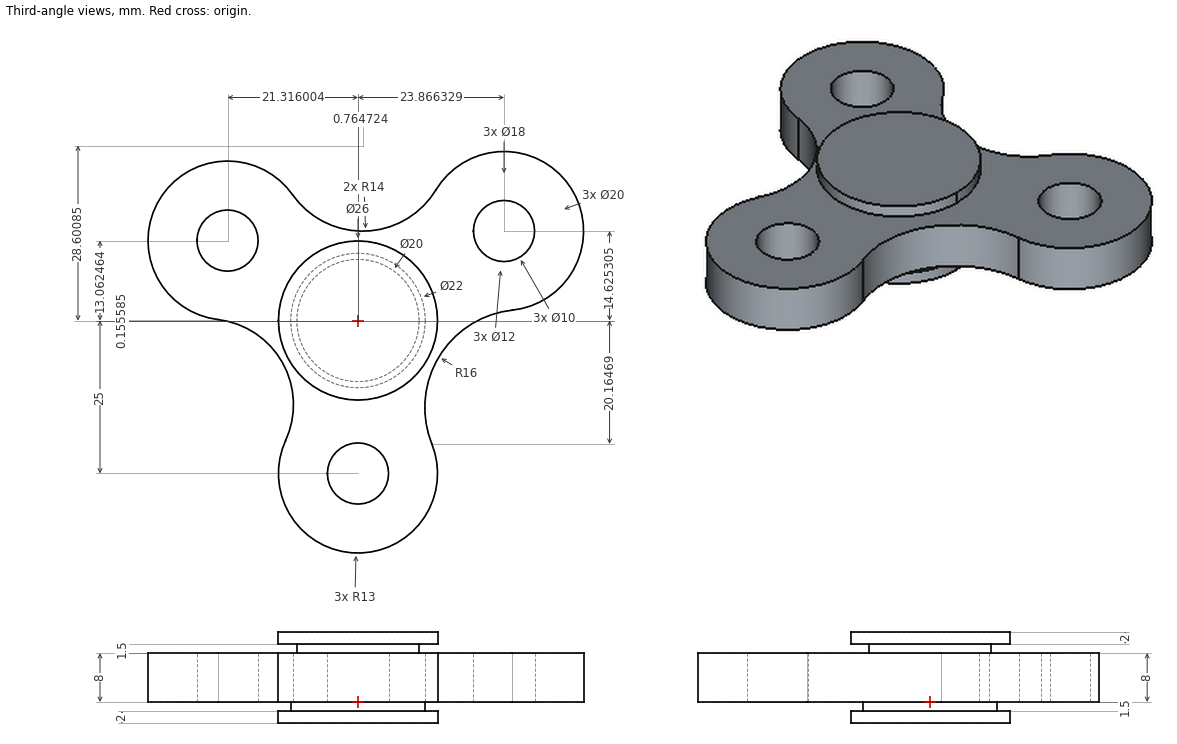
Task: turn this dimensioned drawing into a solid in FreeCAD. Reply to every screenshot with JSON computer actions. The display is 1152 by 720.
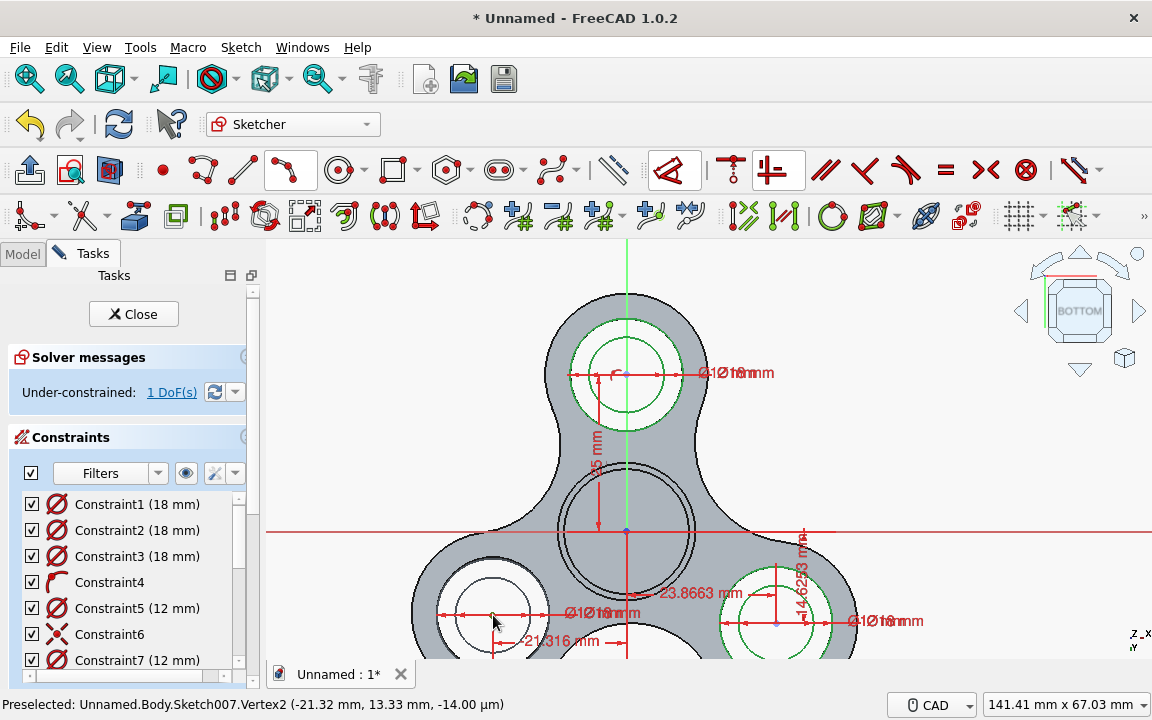
{"action": "key", "text": "i"}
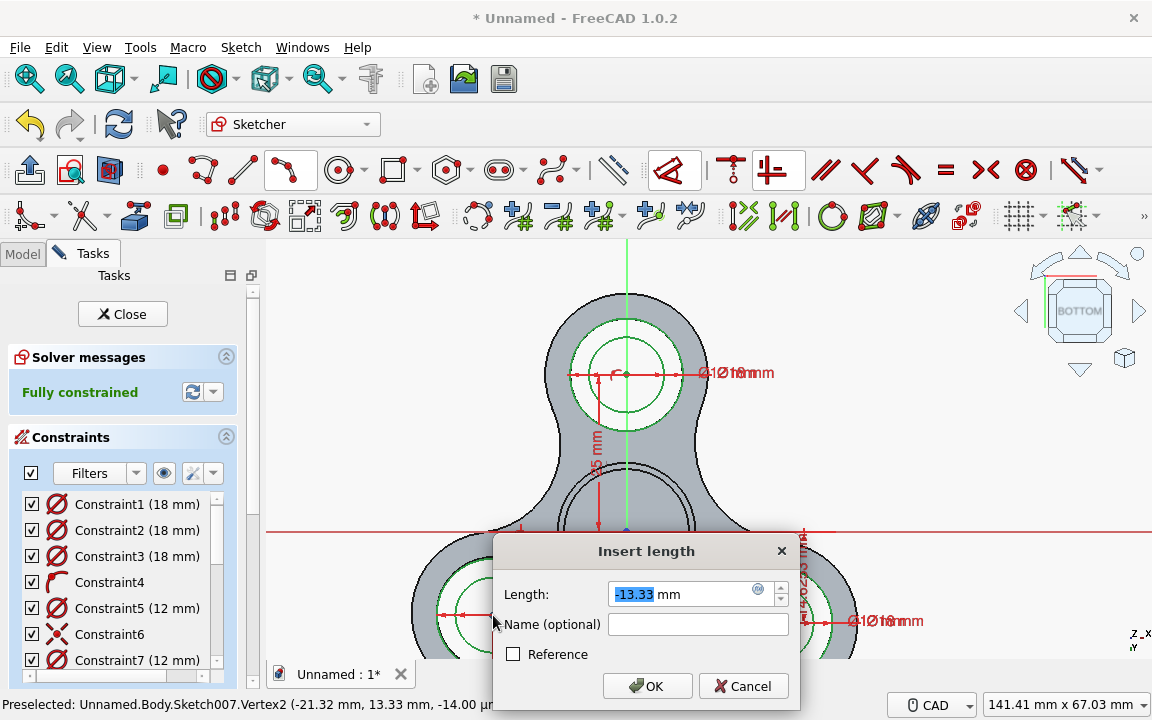
{"action": "type", "text": "-13.062464"}
{"action": "key", "text": "Return"}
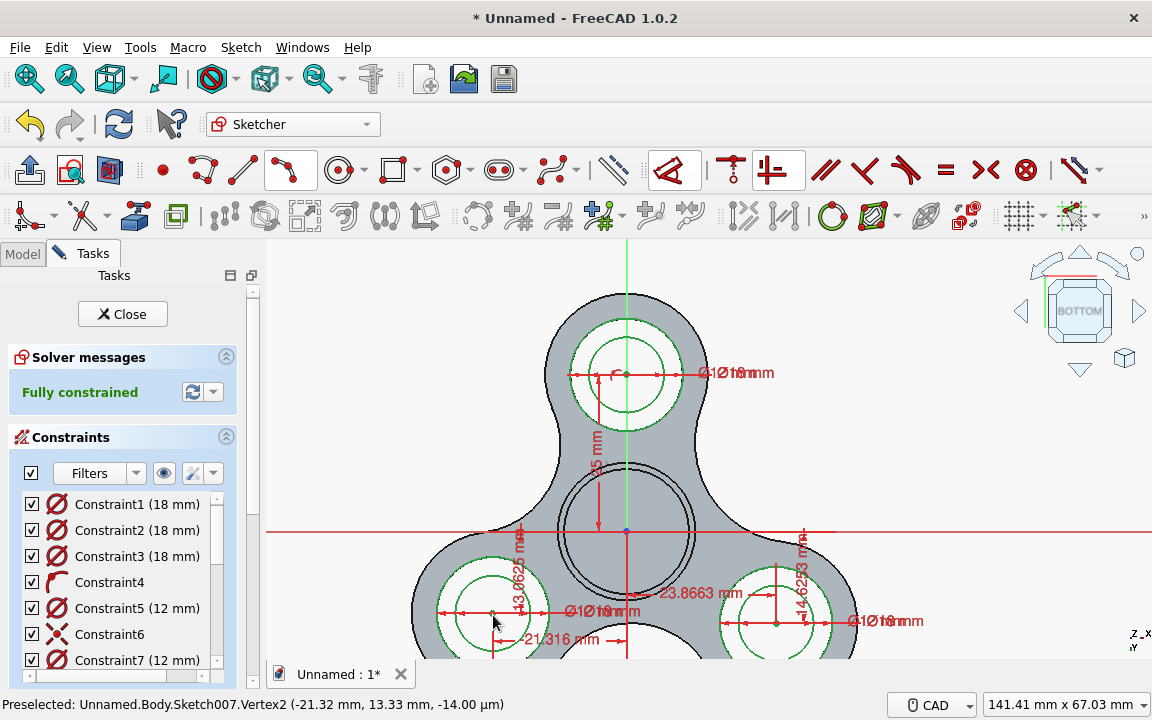
{"action": "left_click", "coordinate": [123, 314]}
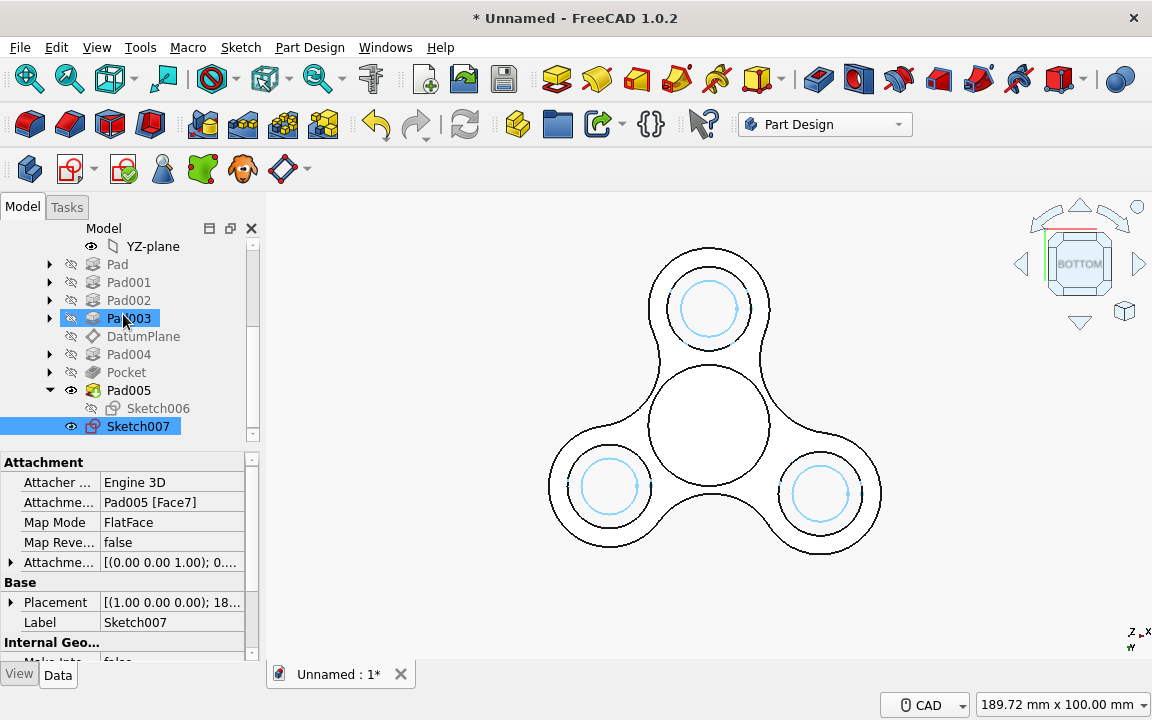
{"action": "left_click", "coordinate": [558, 80]}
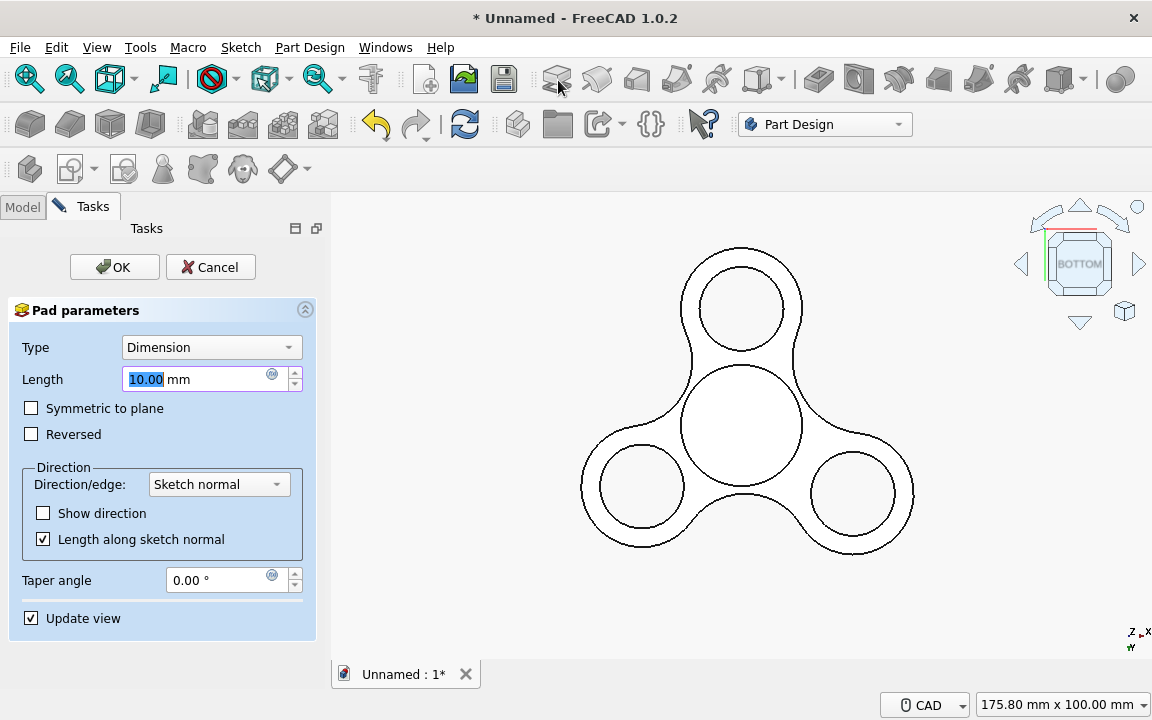
{"action": "type", "text": "8"}
{"action": "key", "text": "Tab"}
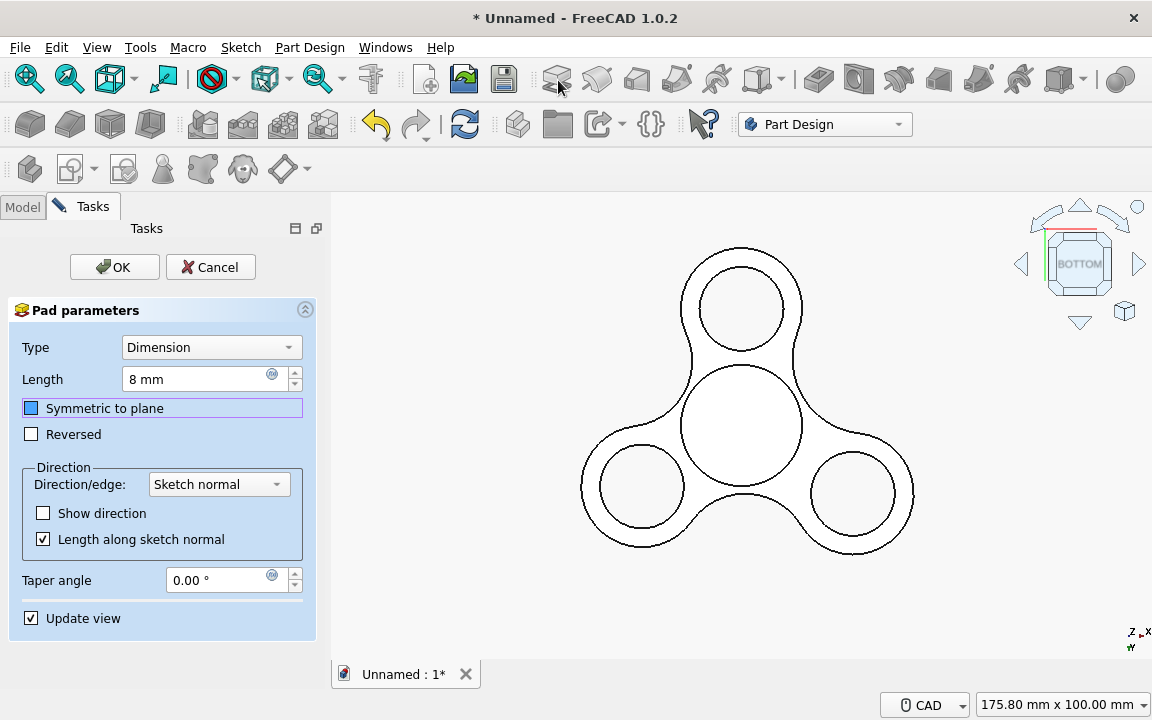
{"action": "left_click", "coordinate": [30, 434]}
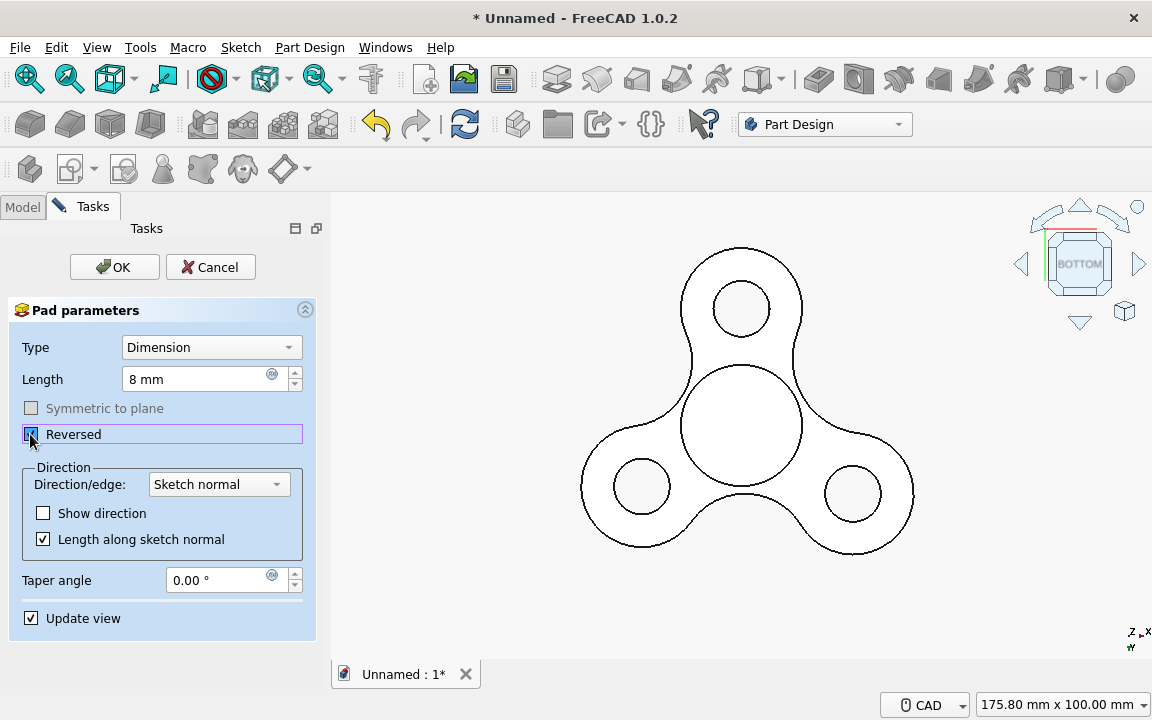
{"action": "left_click", "coordinate": [115, 267]}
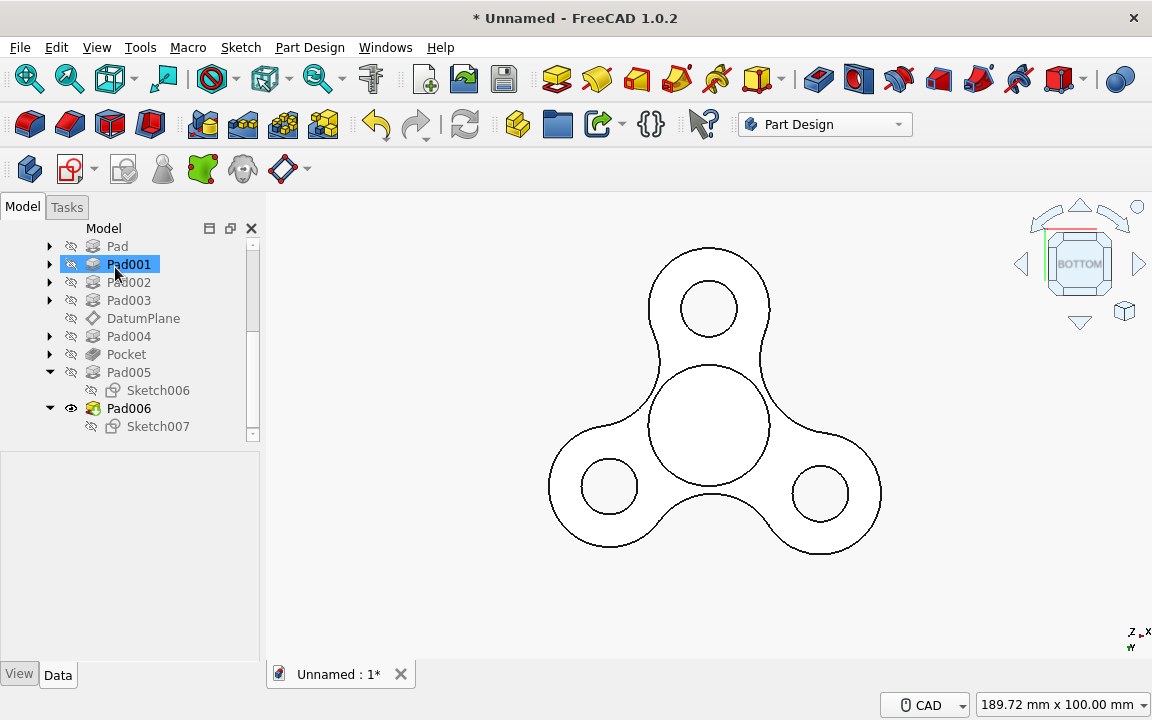
{"action": "left_click", "coordinate": [762, 488]}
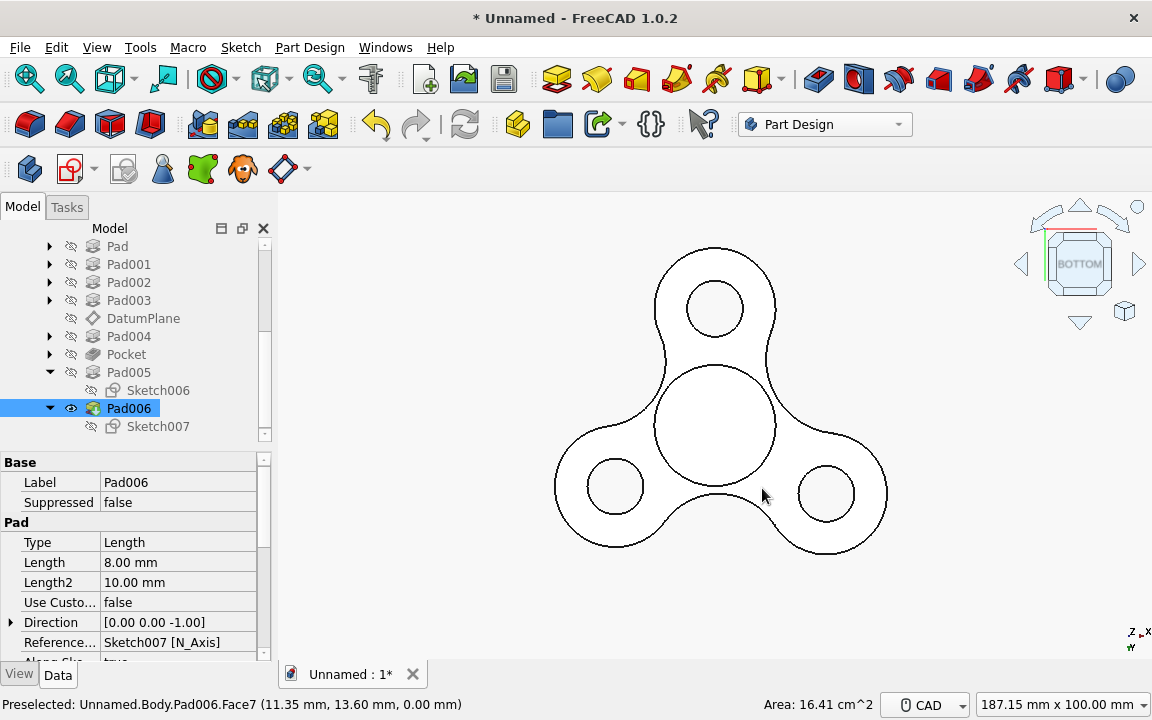
{"action": "left_click", "coordinate": [70, 170]}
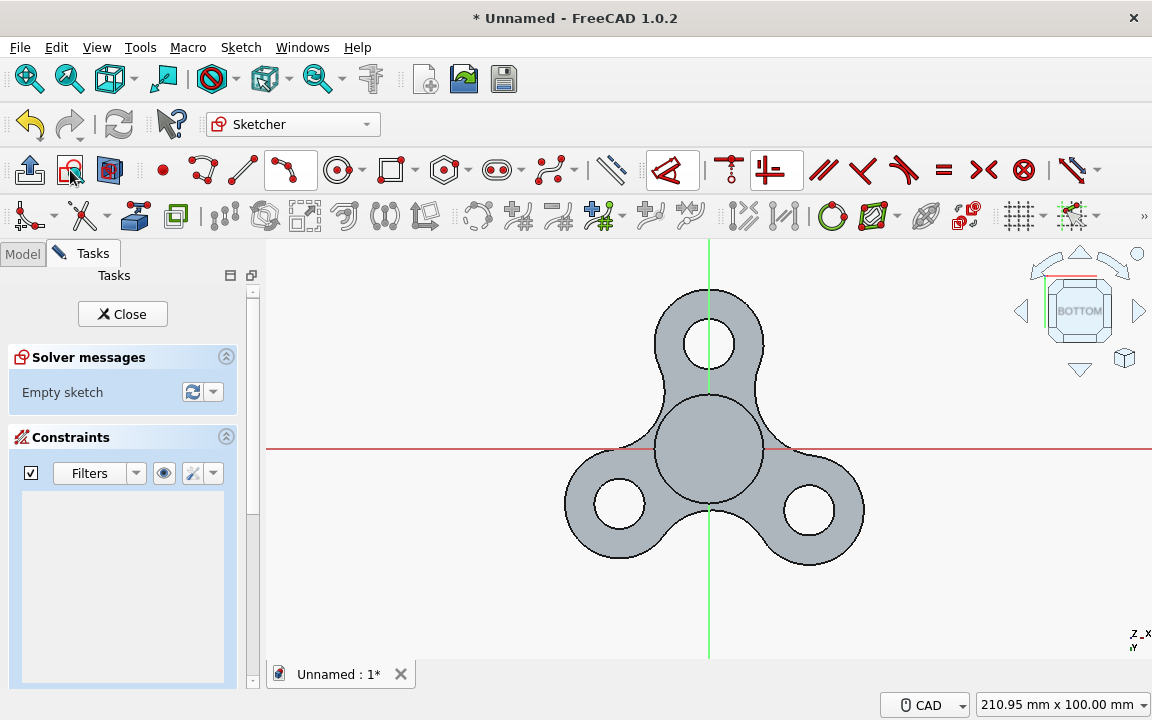
{"action": "left_click", "coordinate": [110, 170]}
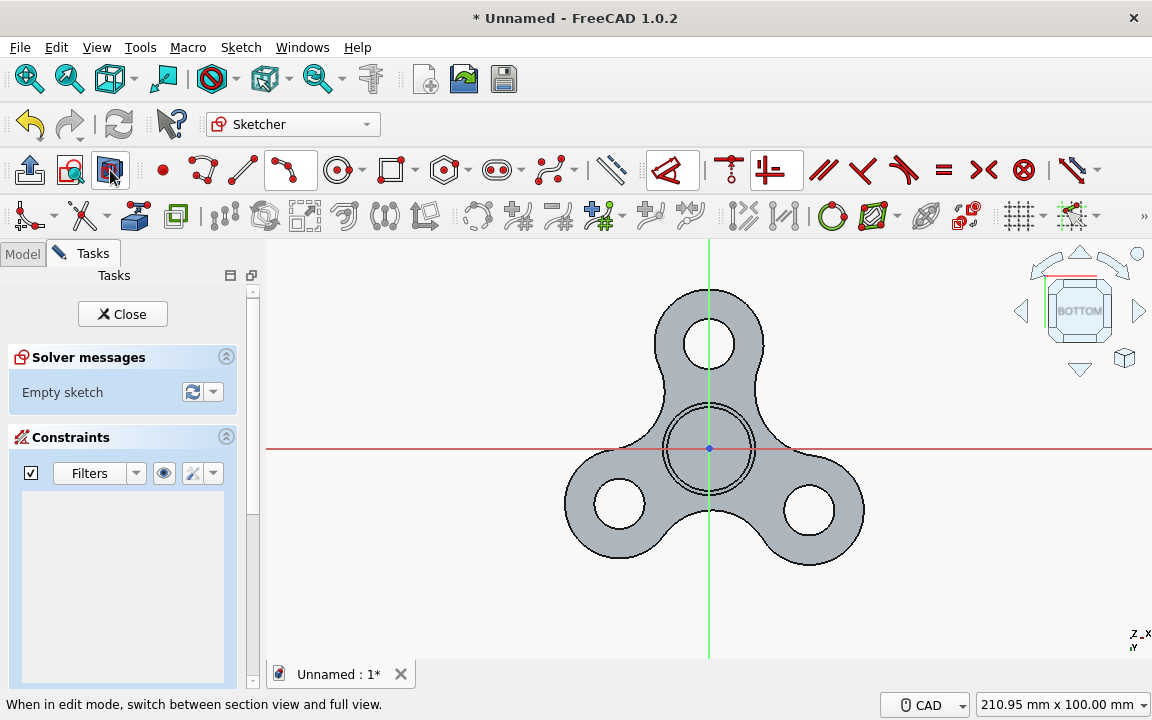
{"action": "left_click", "coordinate": [338, 170]}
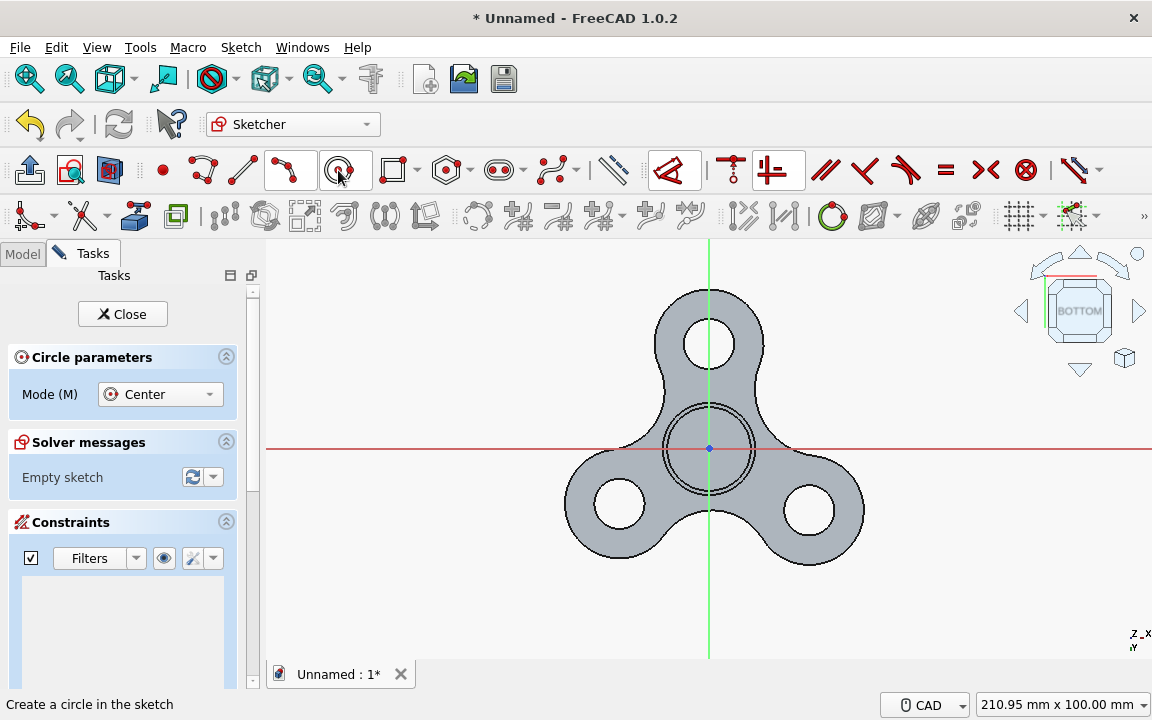
{"action": "left_click", "coordinate": [809, 510]}
{"action": "mouse_move", "coordinate": [827, 493]}